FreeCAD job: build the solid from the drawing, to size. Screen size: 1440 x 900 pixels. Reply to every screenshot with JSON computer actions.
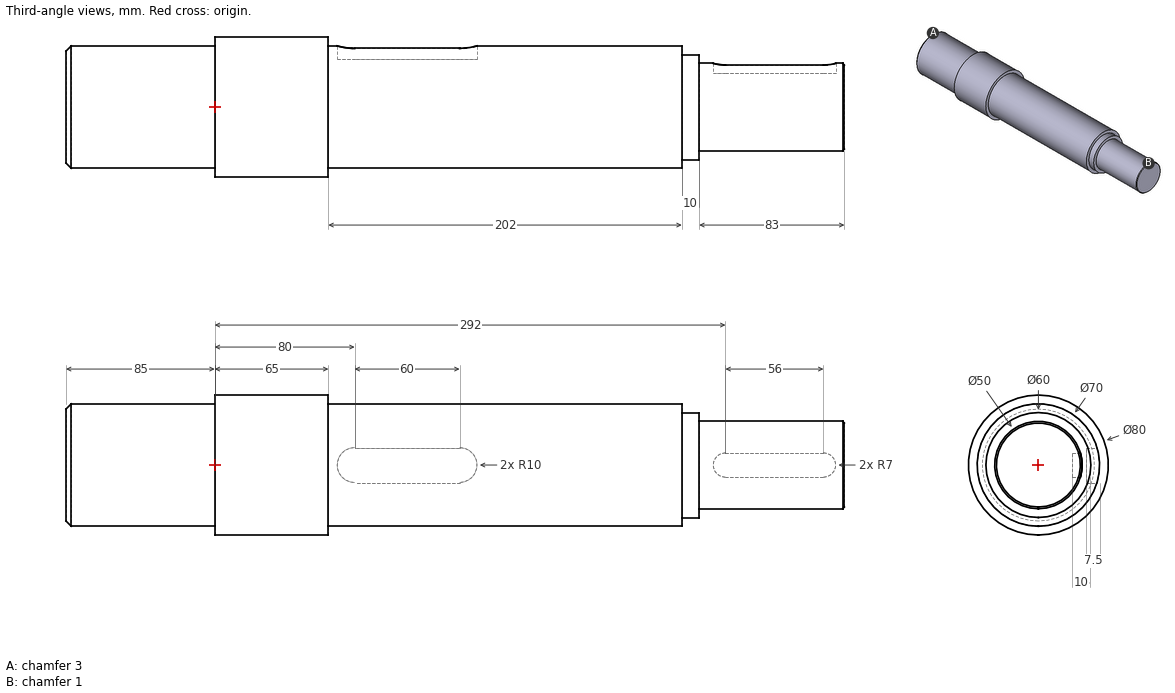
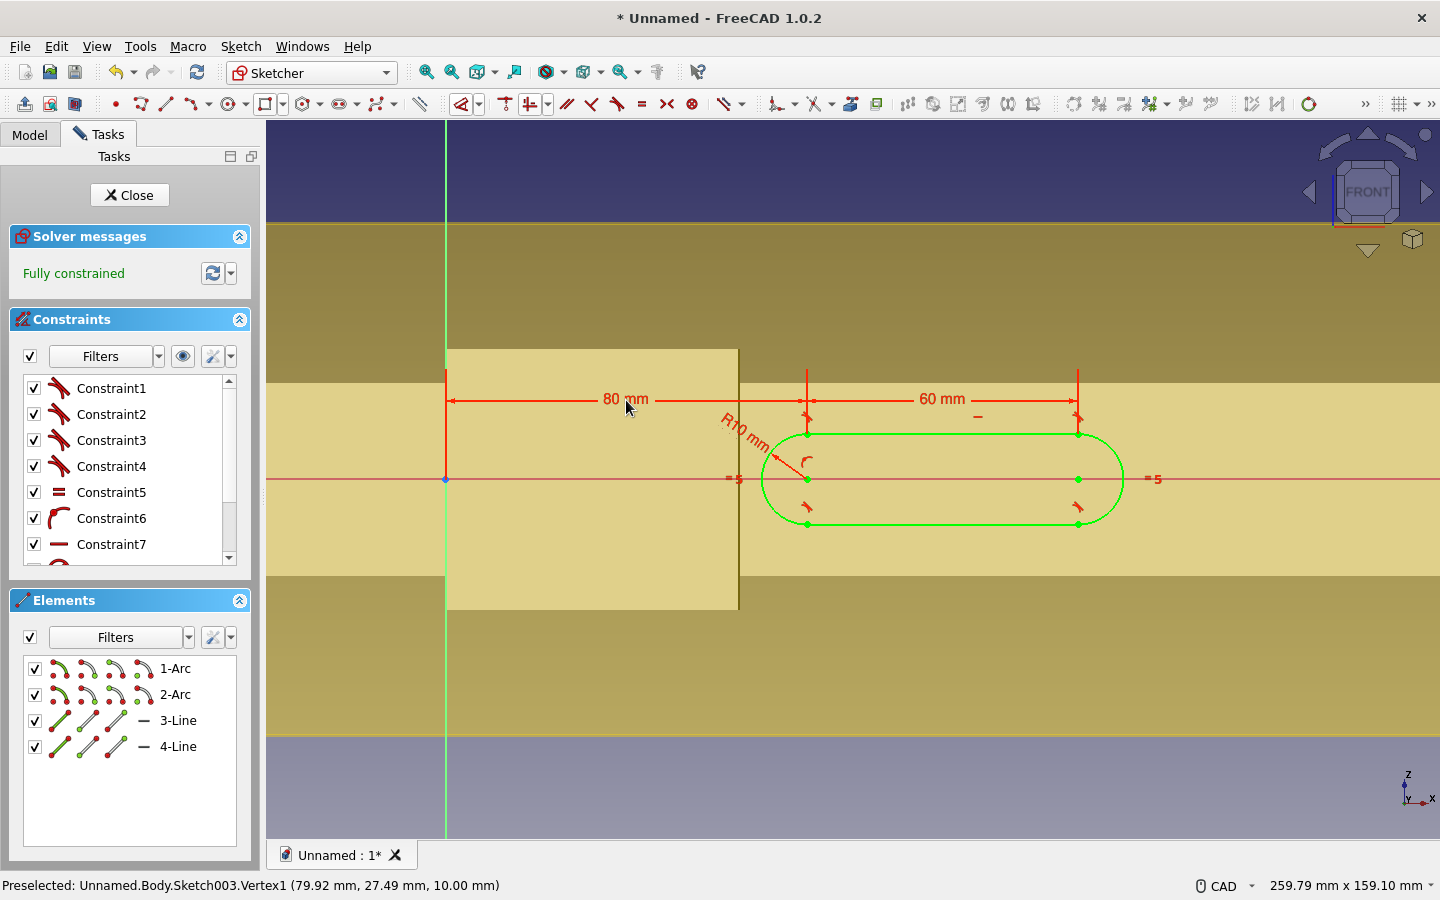
{"action": "left_click", "coordinate": [130, 195]}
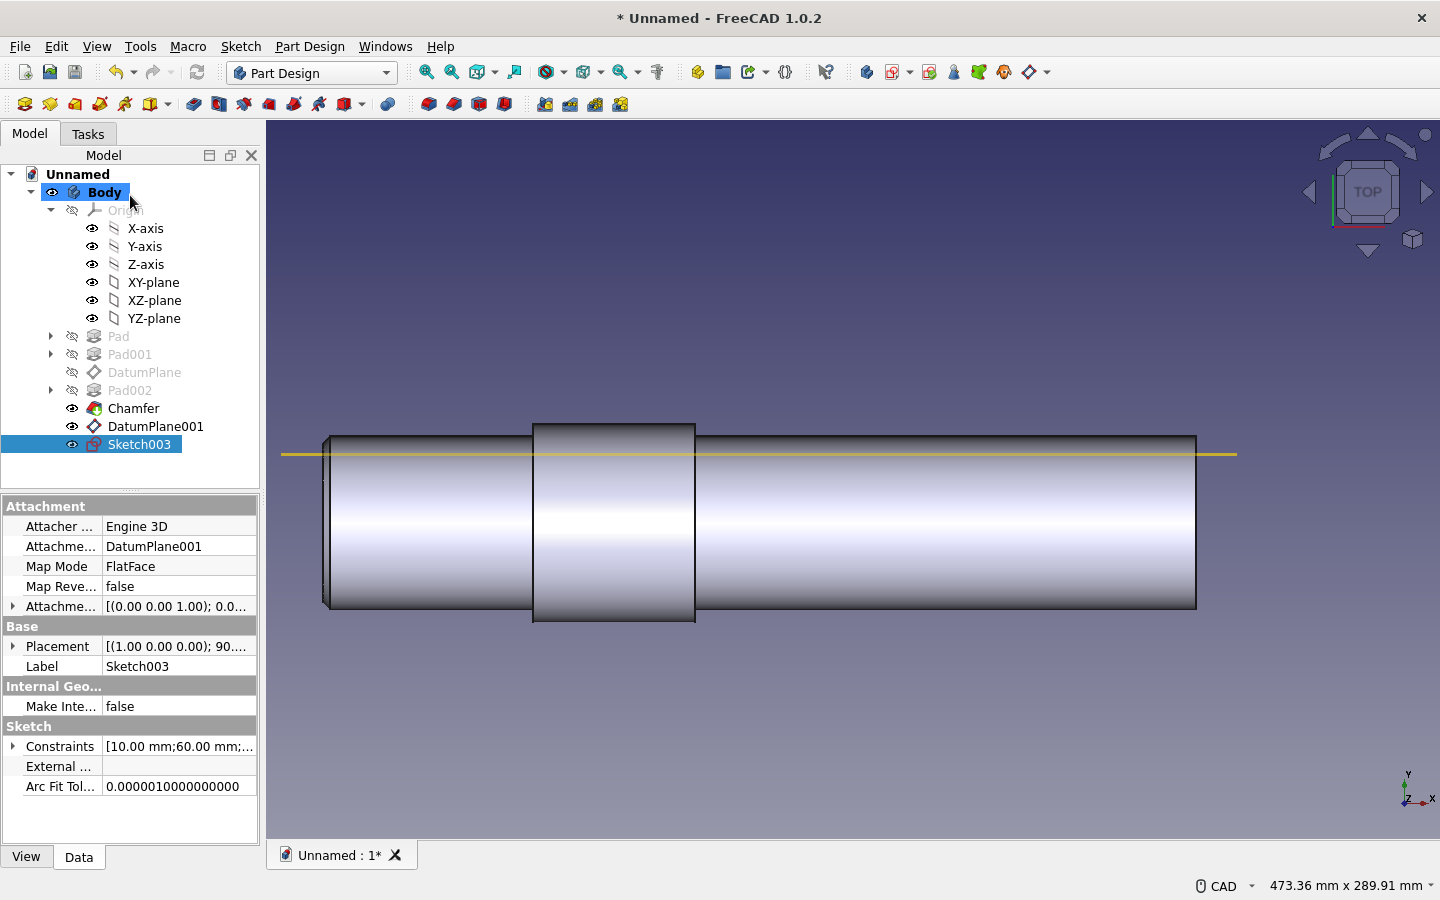
{"action": "left_click", "coordinate": [194, 104]}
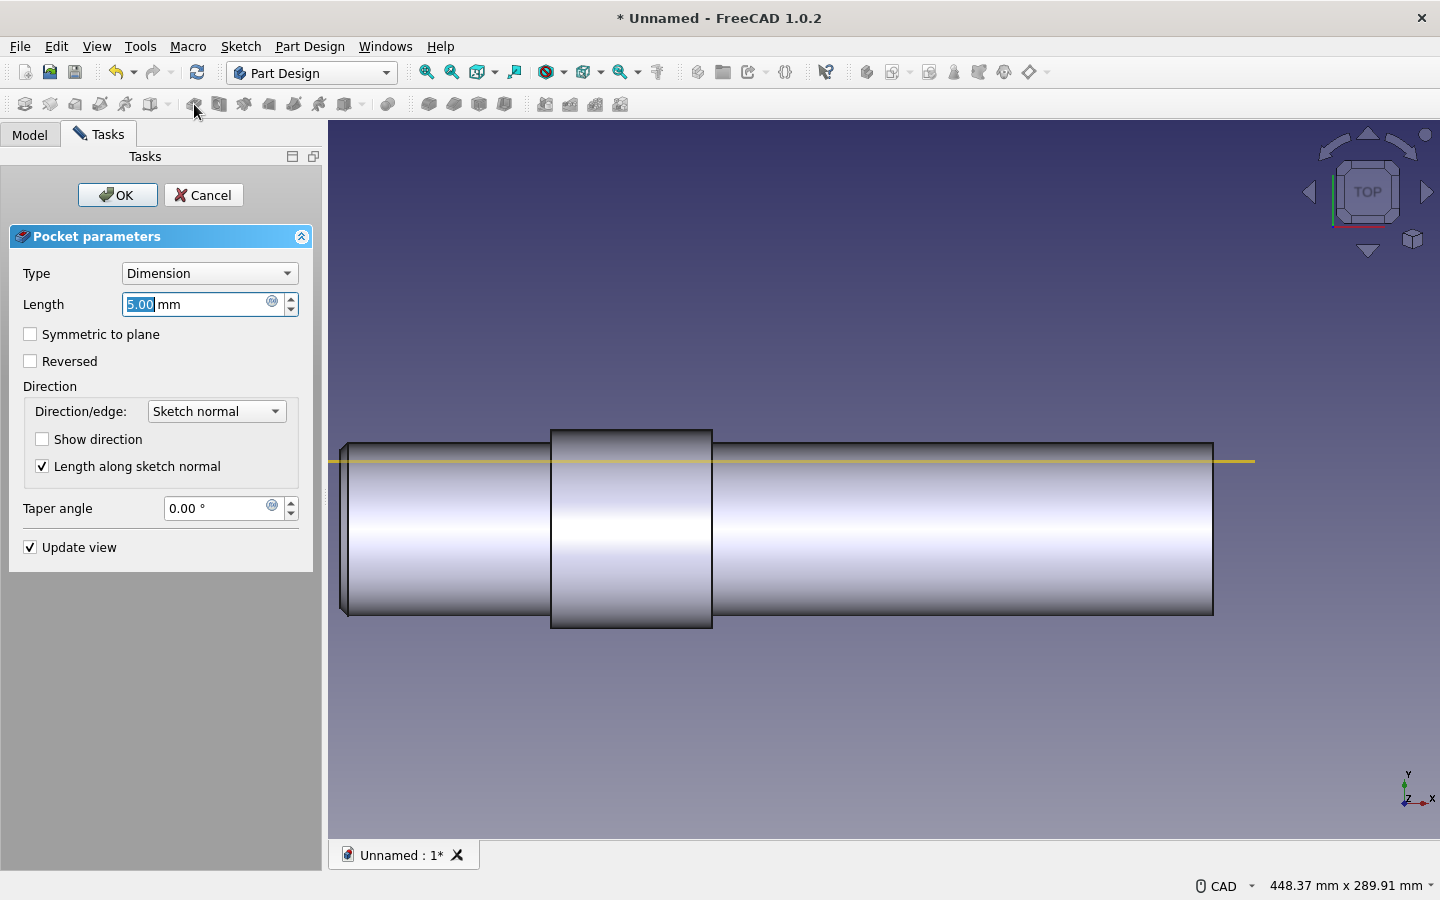
{"action": "type", "text": "7.5"}
{"action": "key", "text": "Tab"}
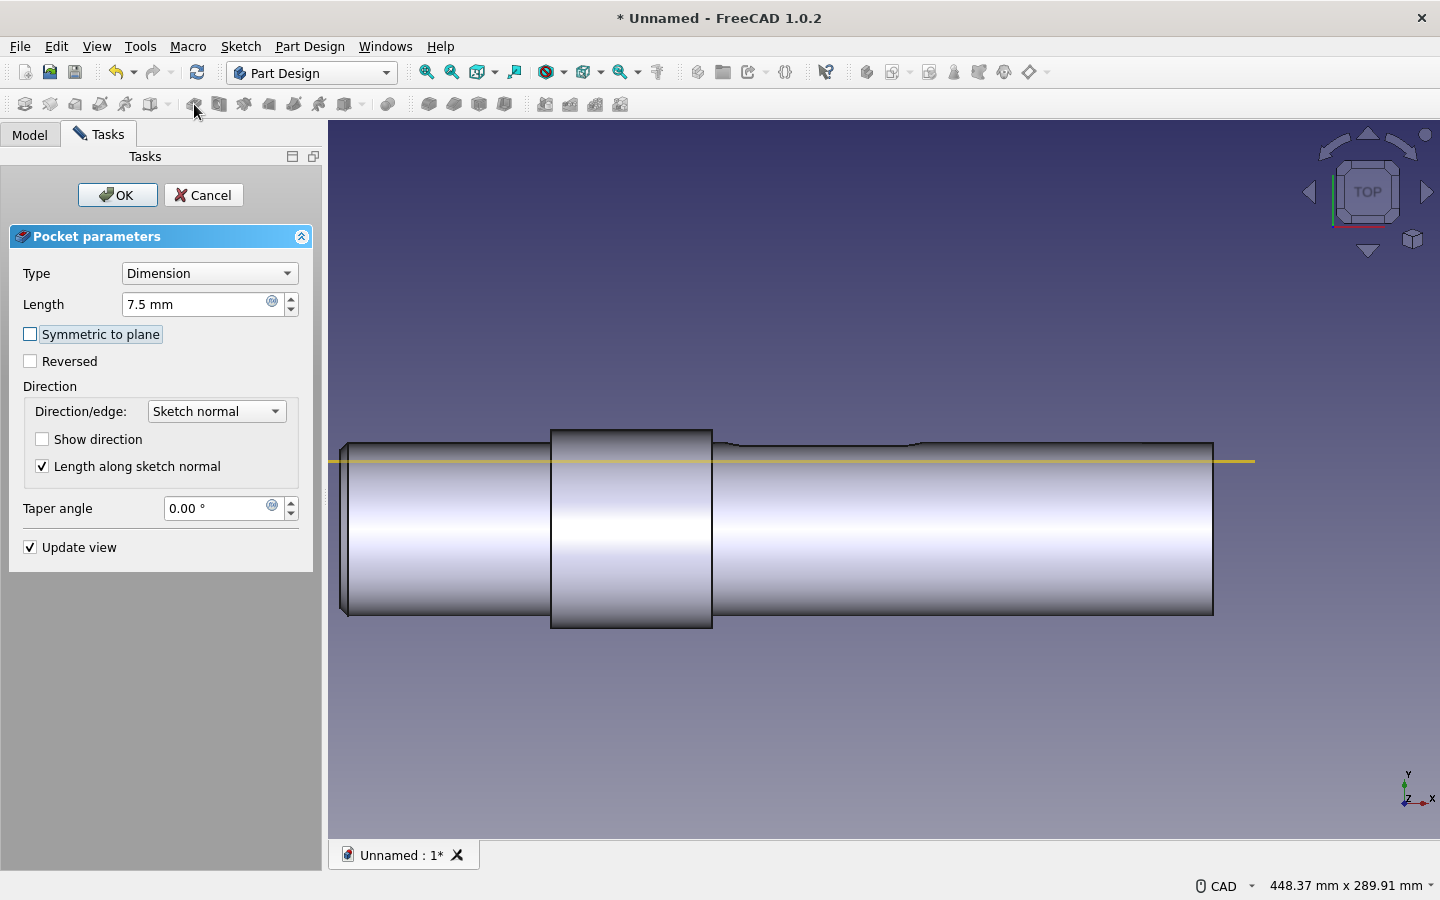
{"action": "left_click", "coordinate": [118, 195]}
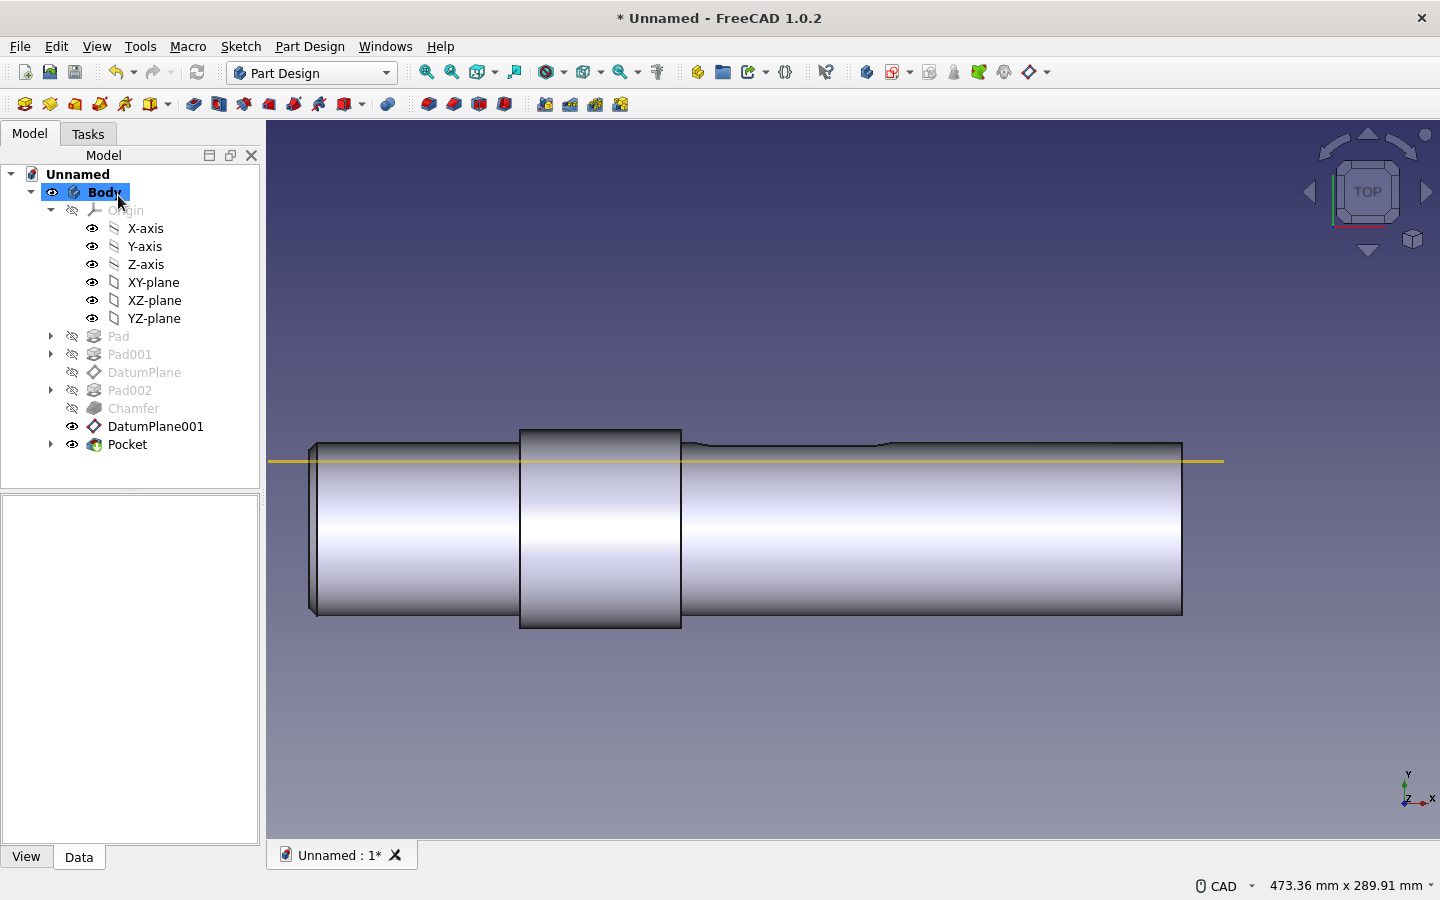
{"action": "left_click", "coordinate": [117, 426]}
{"action": "key", "text": "space"}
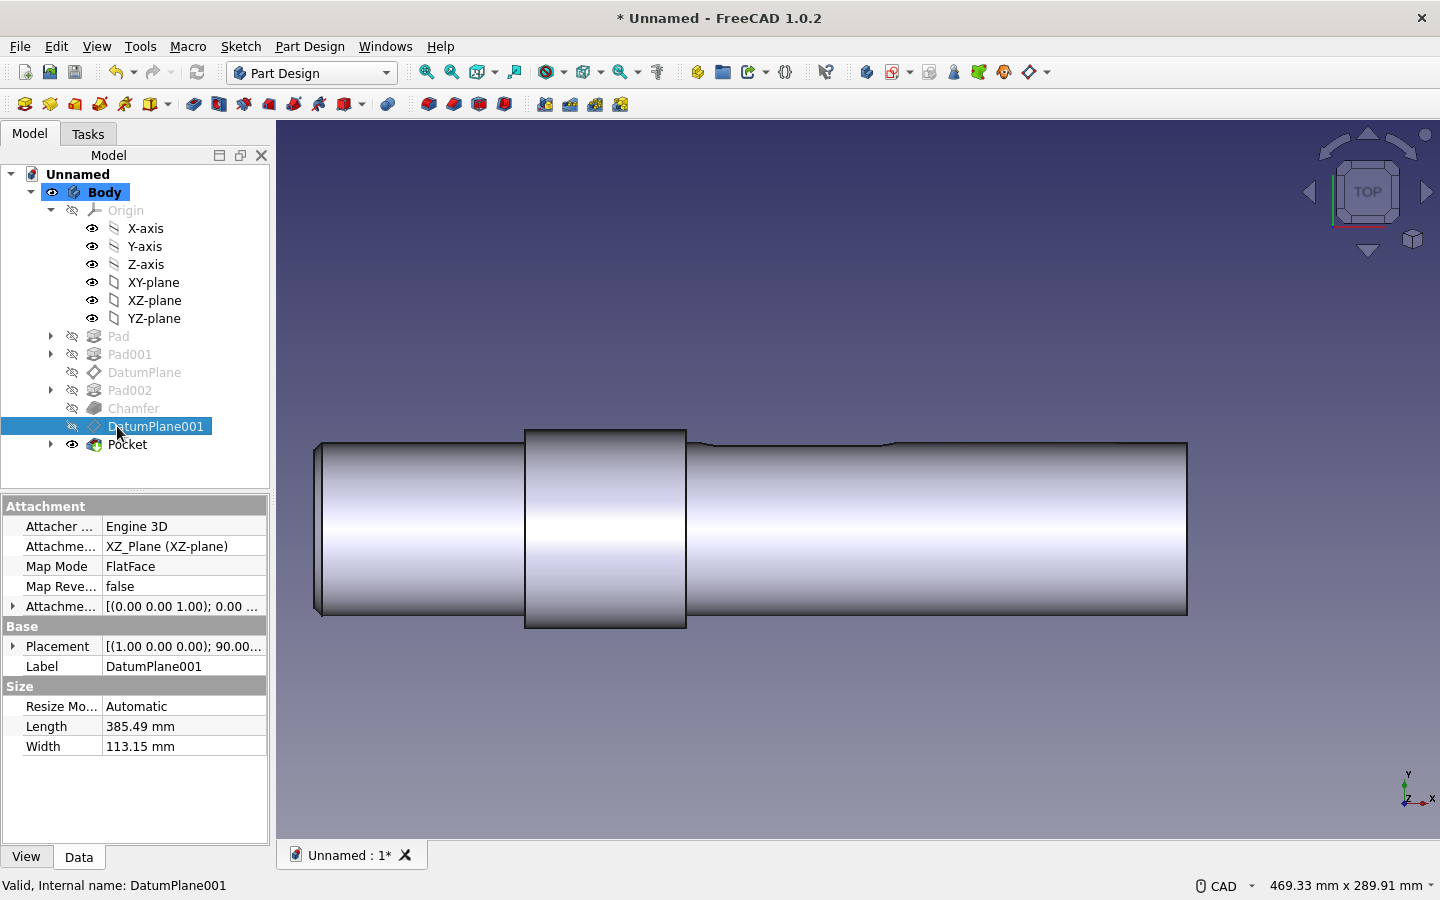
{"action": "key", "text": "0"}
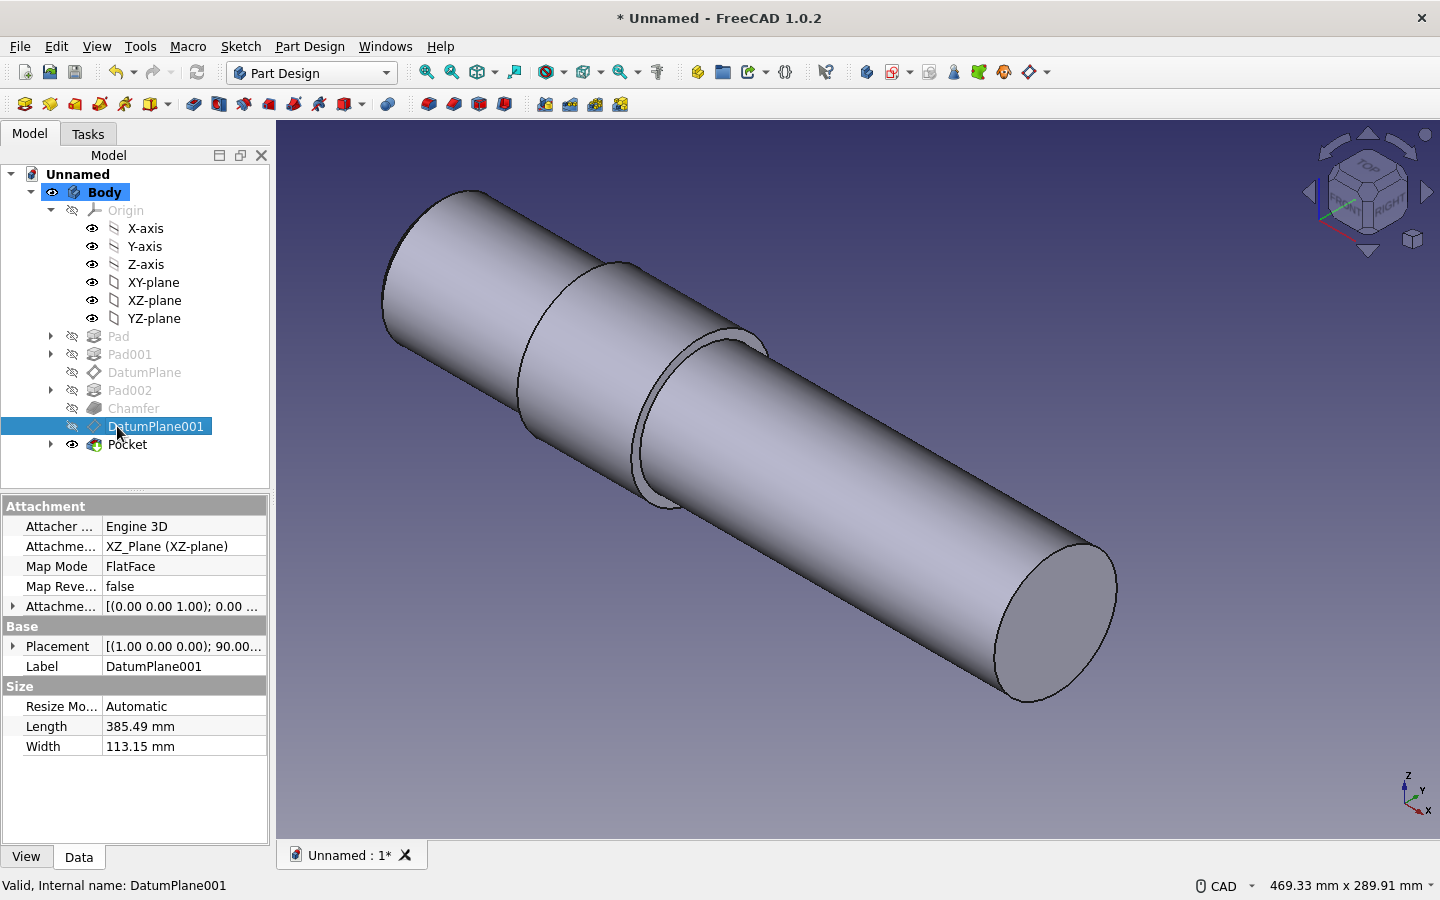
{"action": "left_click", "coordinate": [1056, 622]}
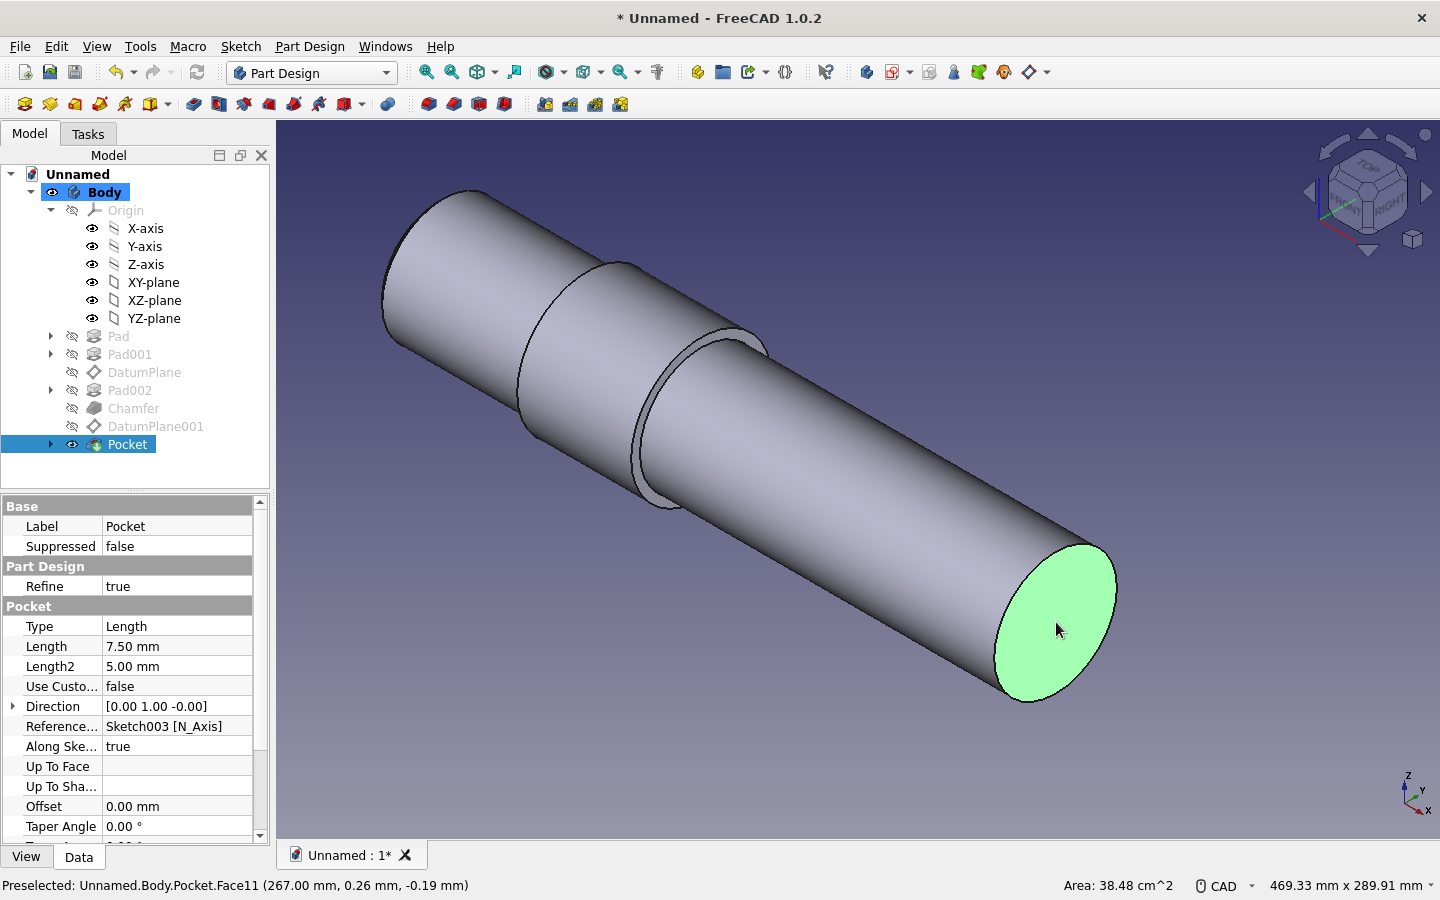
{"action": "left_click", "coordinate": [892, 72]}